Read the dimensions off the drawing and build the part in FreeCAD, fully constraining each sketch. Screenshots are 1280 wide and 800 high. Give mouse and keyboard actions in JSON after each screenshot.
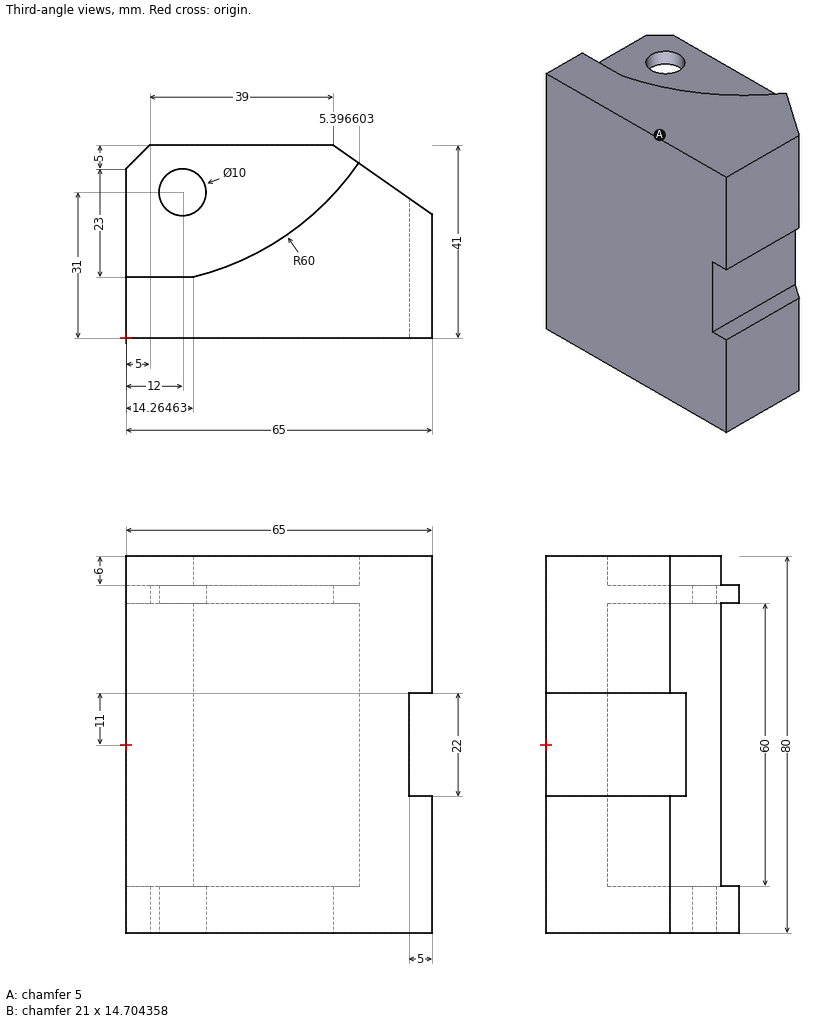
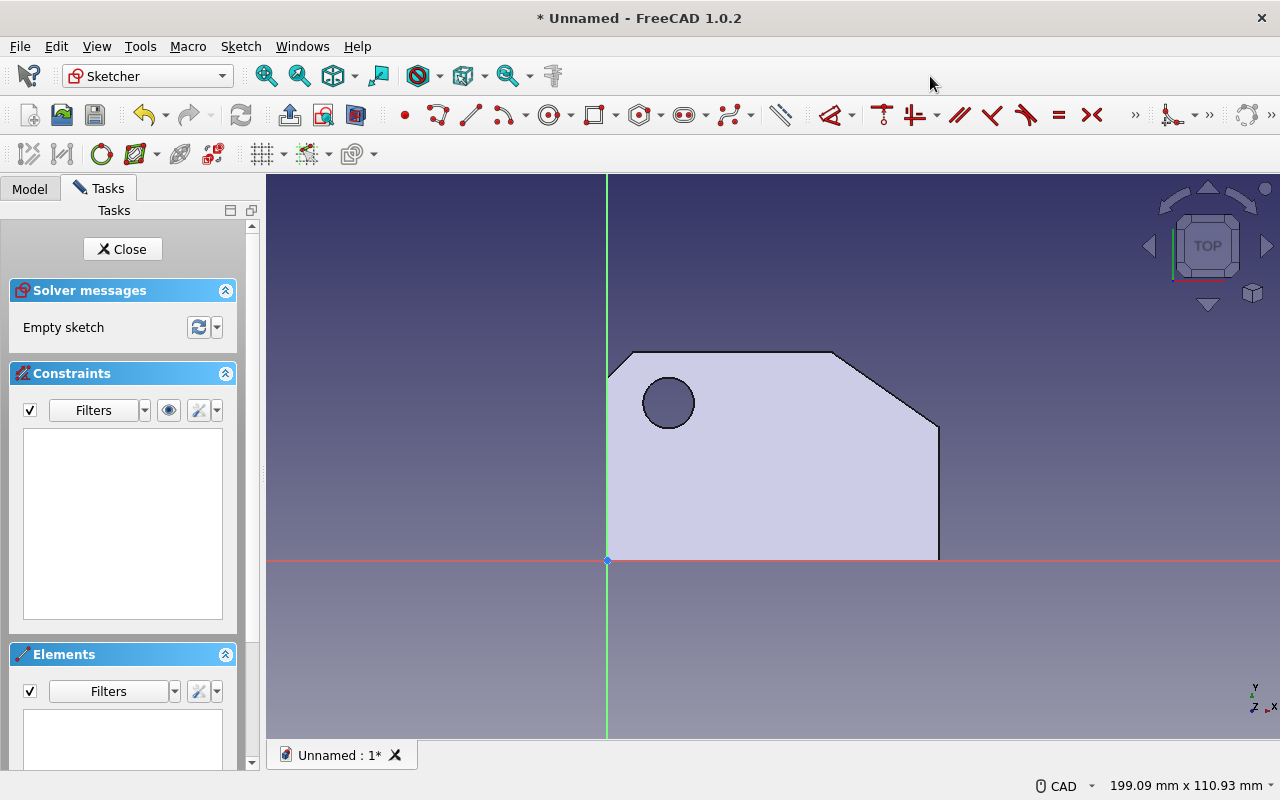
{"action": "scroll", "coordinate": [768, 457], "scroll_direction": "up", "scroll_amount": 3}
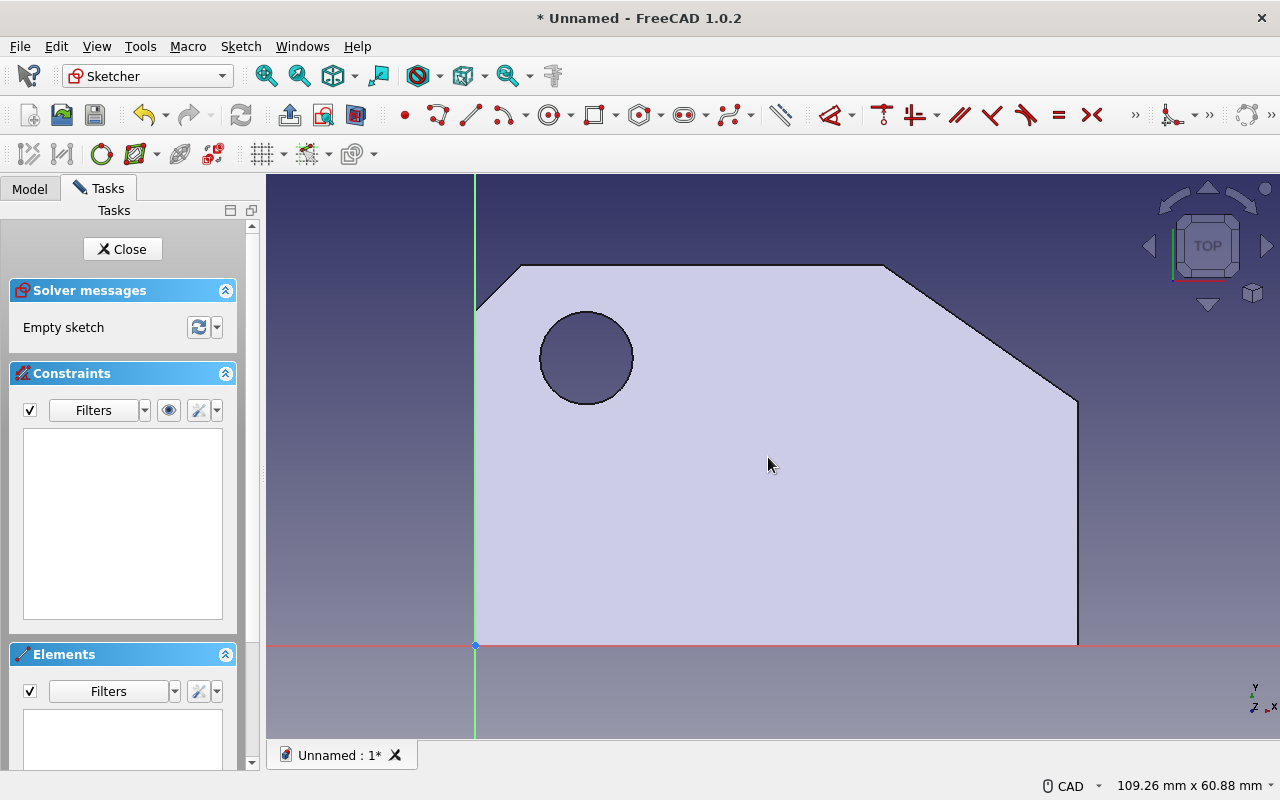
{"action": "key", "text": "g m"}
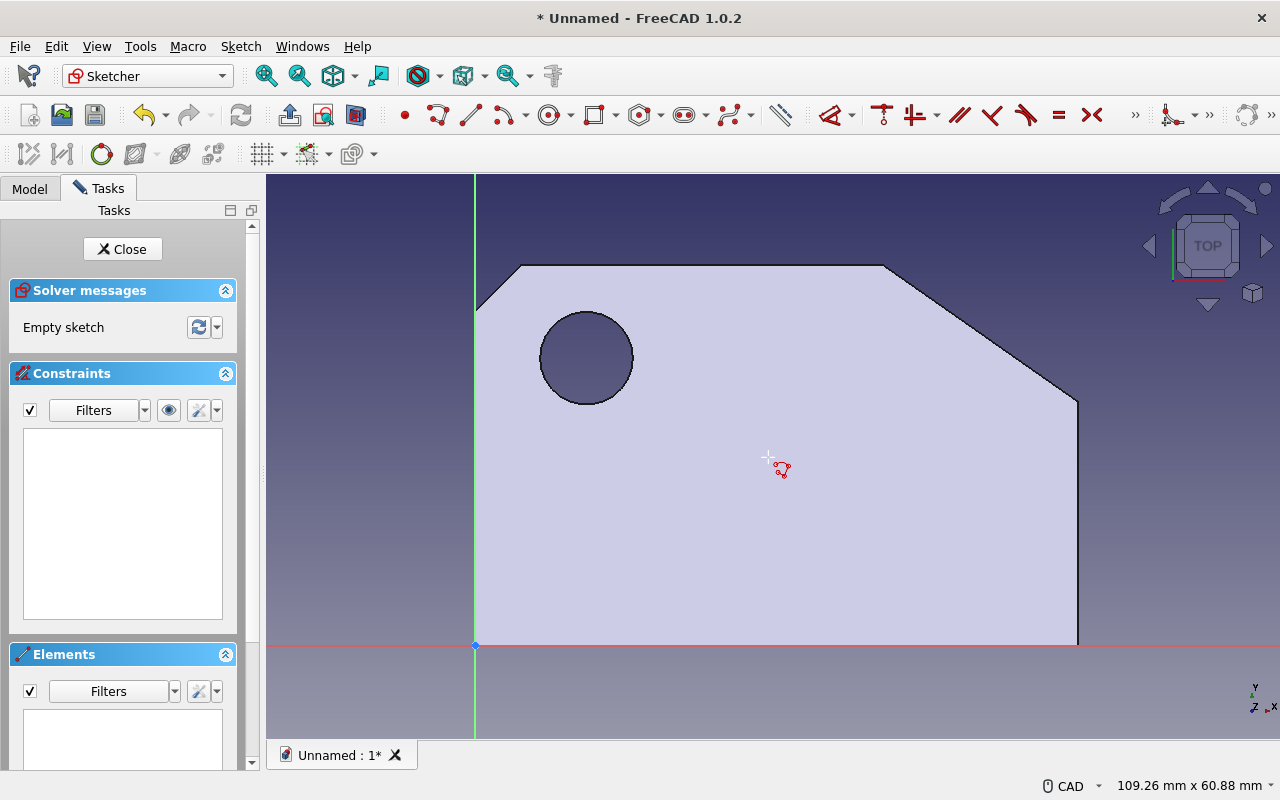
{"action": "left_click", "coordinate": [934, 300]}
{"action": "left_click", "coordinate": [883, 265]}
{"action": "left_click", "coordinate": [521, 265]}
{"action": "left_click", "coordinate": [475, 312]}
{"action": "left_click", "coordinate": [484, 525]}
{"action": "left_click", "coordinate": [607, 525]}
{"action": "right_click", "coordinate": [607, 525]}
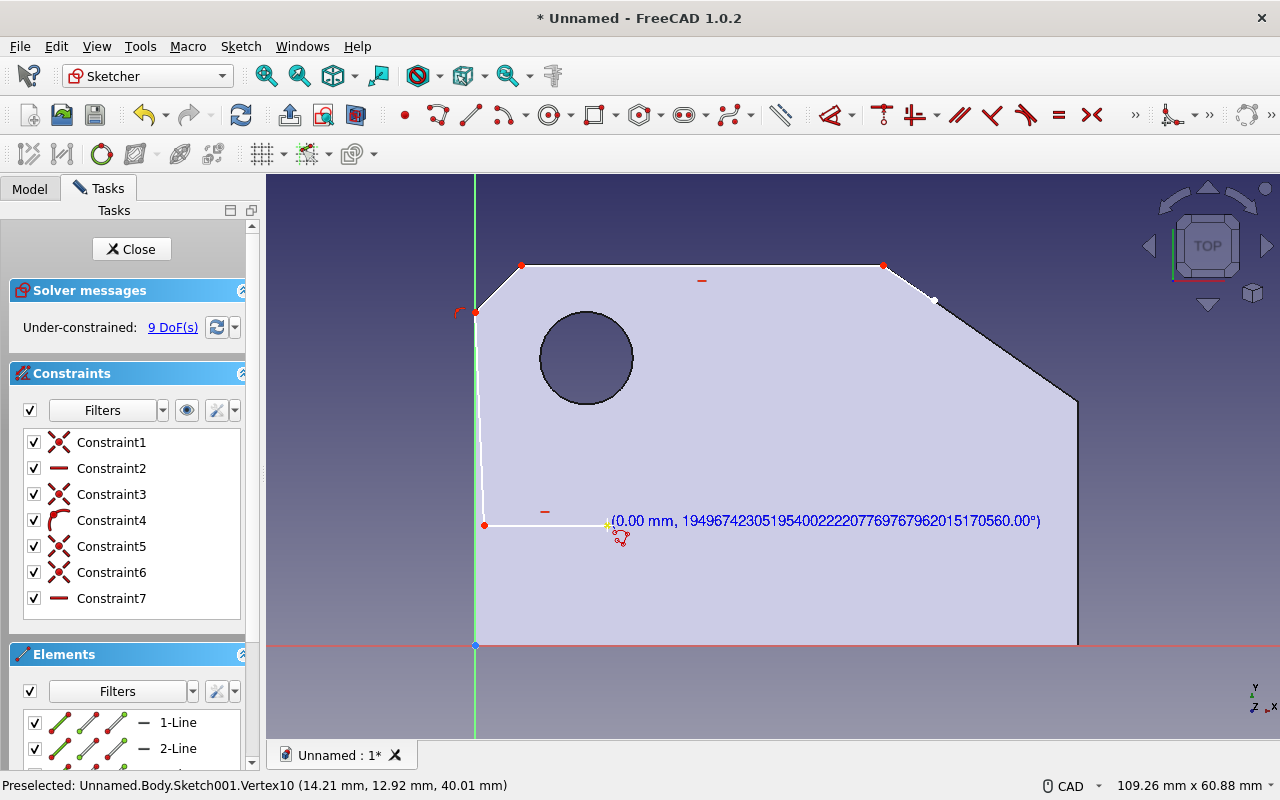
{"action": "key", "text": "g 3 a"}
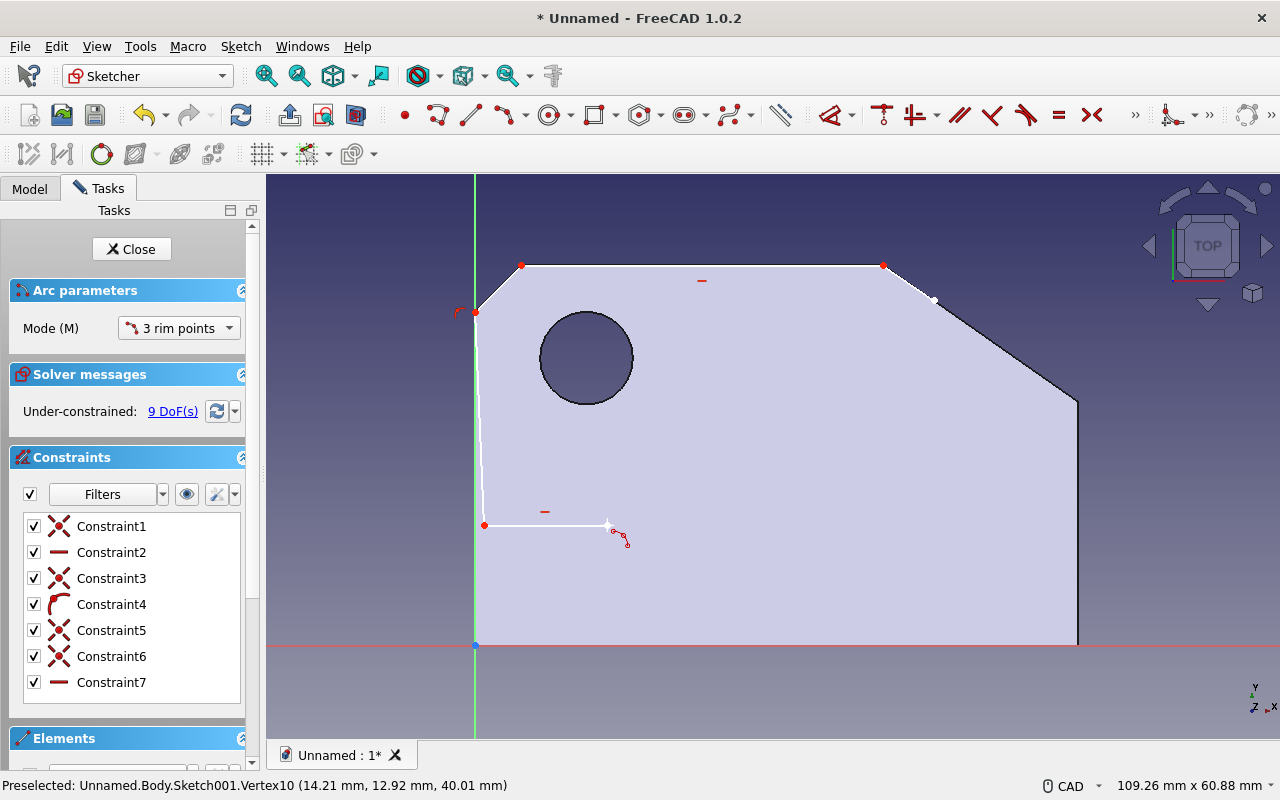
{"action": "left_click", "coordinate": [607, 526]}
{"action": "left_click", "coordinate": [934, 301]}
{"action": "left_click", "coordinate": [791, 443]}
{"action": "key", "text": "Escape"}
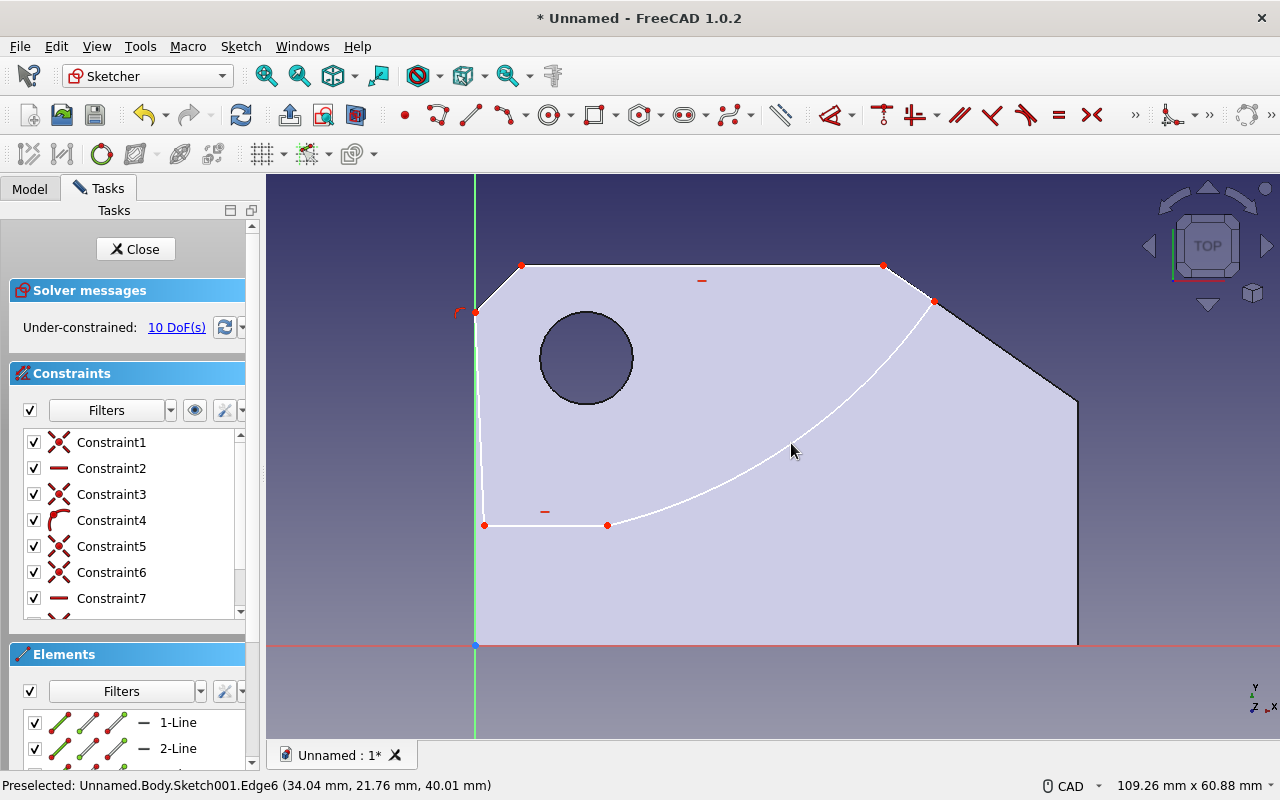
{"action": "left_click", "coordinate": [478, 377]}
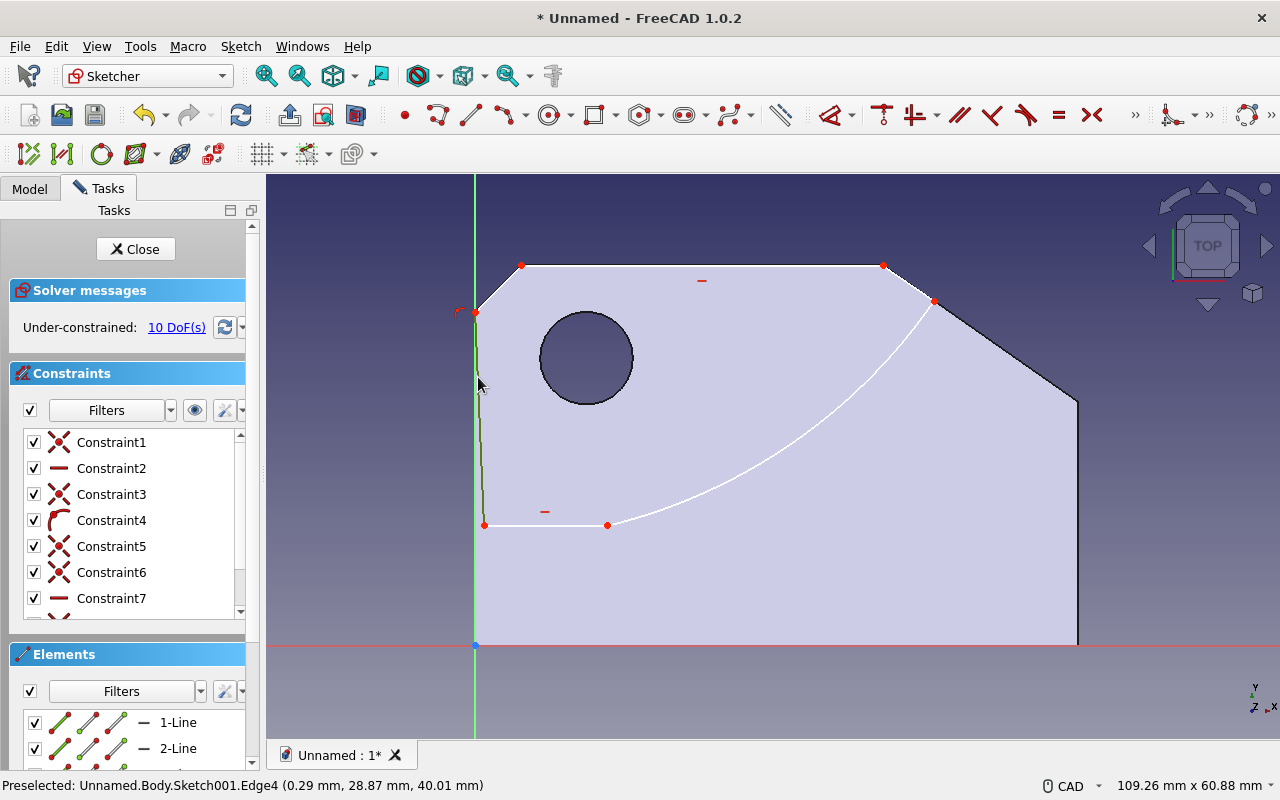
{"action": "key", "text": "v"}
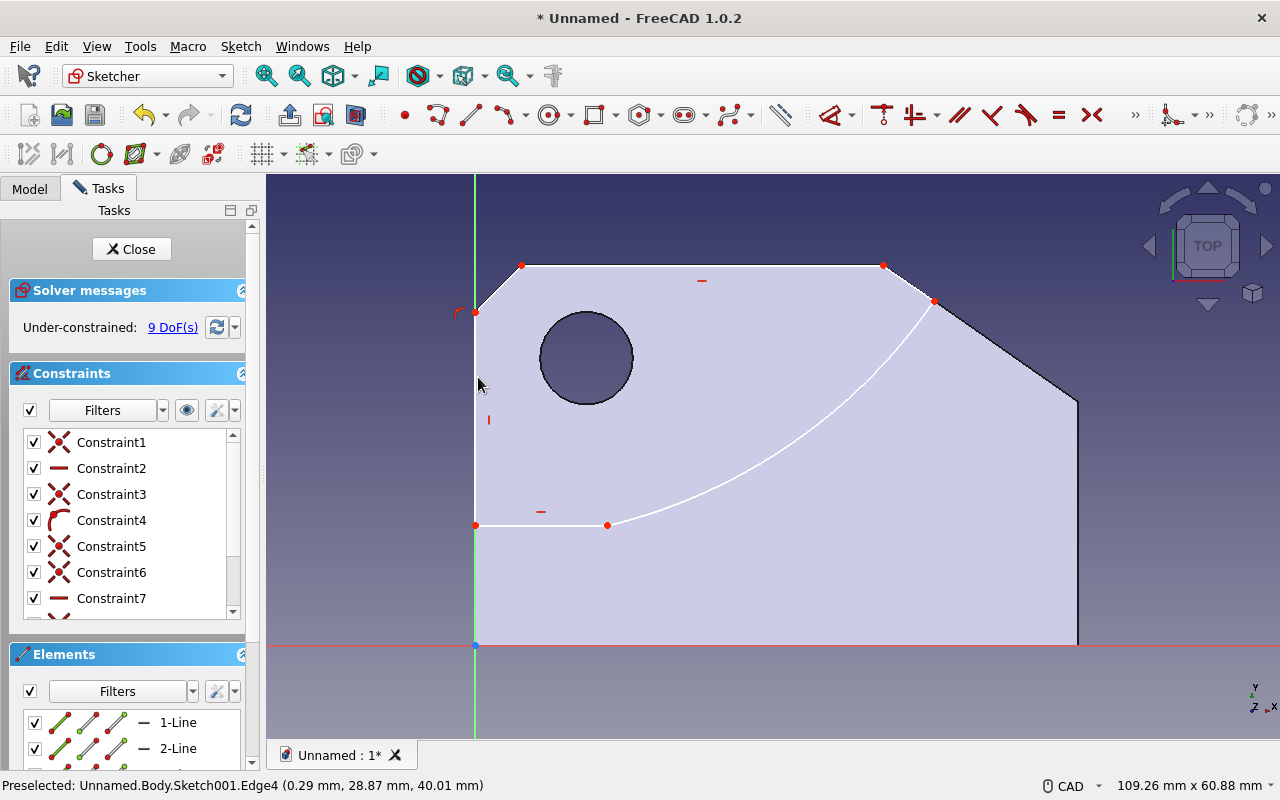
{"action": "scroll", "coordinate": [705, 627], "scroll_direction": "down", "scroll_amount": 3}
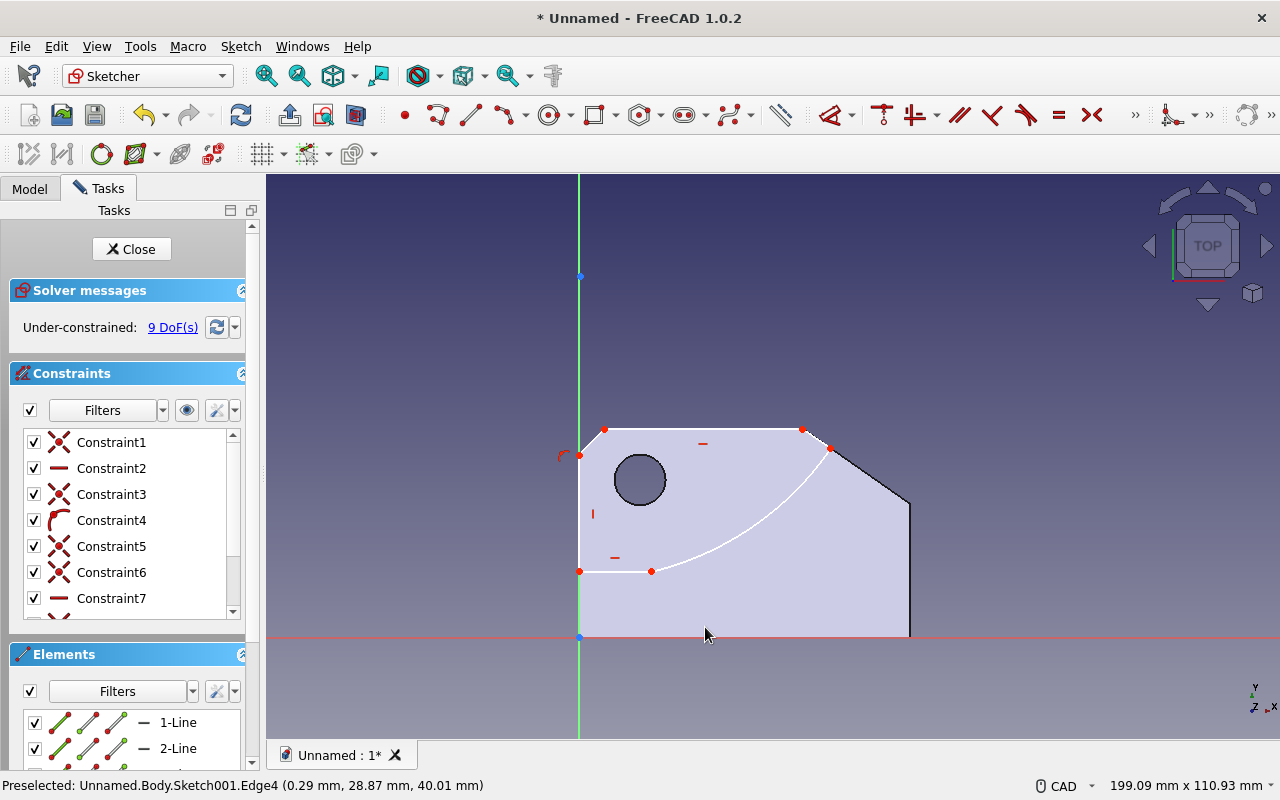
{"action": "left_click", "coordinate": [580, 276]}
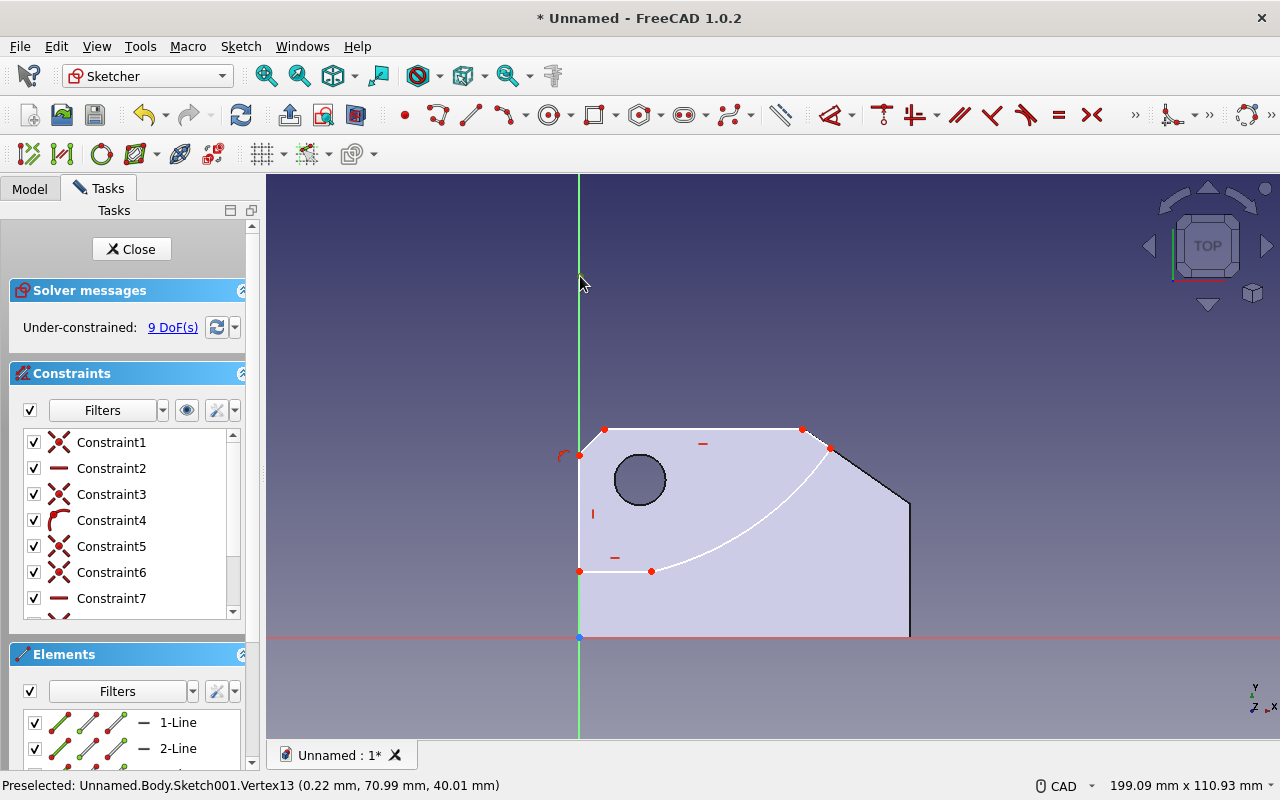
{"action": "left_click", "coordinate": [579, 675]}